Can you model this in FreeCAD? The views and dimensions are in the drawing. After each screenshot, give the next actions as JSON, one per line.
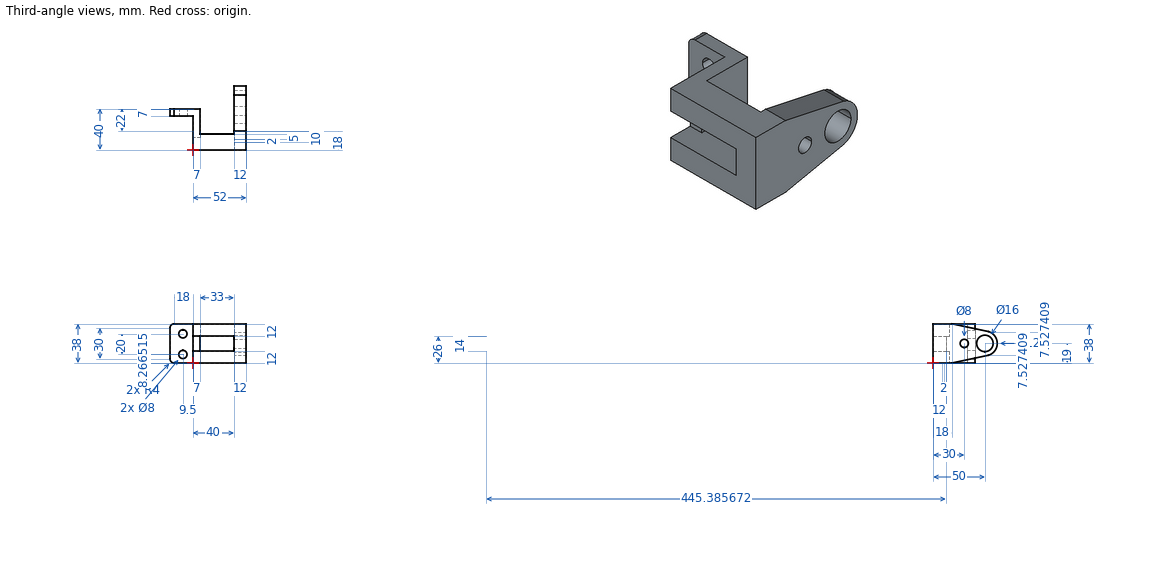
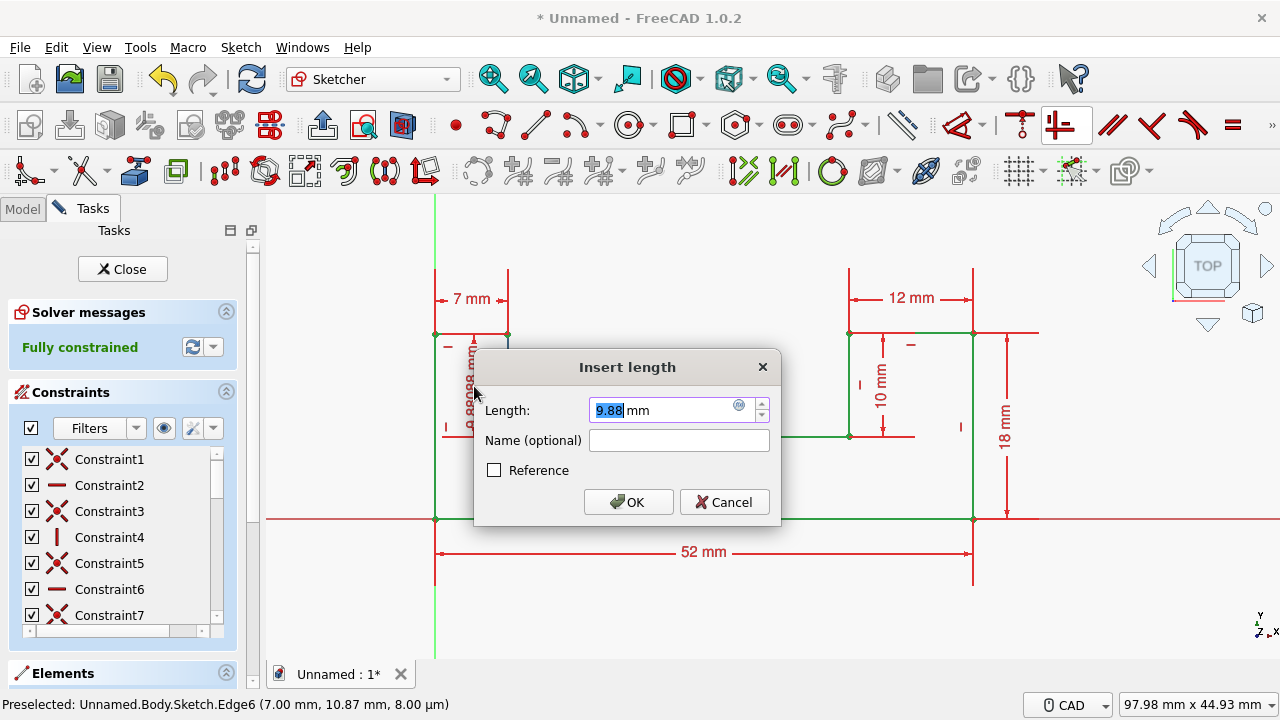
{"action": "type", "text": "10"}
{"action": "key", "text": "Return"}
{"action": "key", "text": "Escape"}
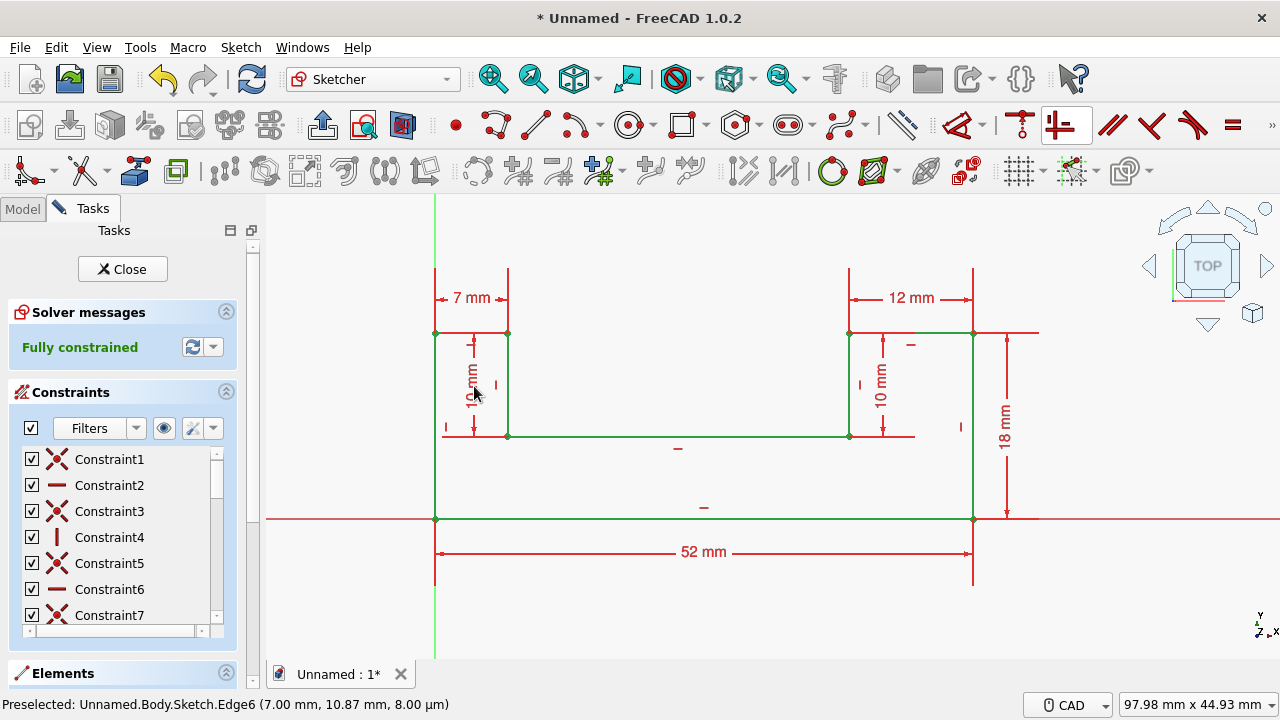
{"action": "left_click", "coordinate": [123, 269]}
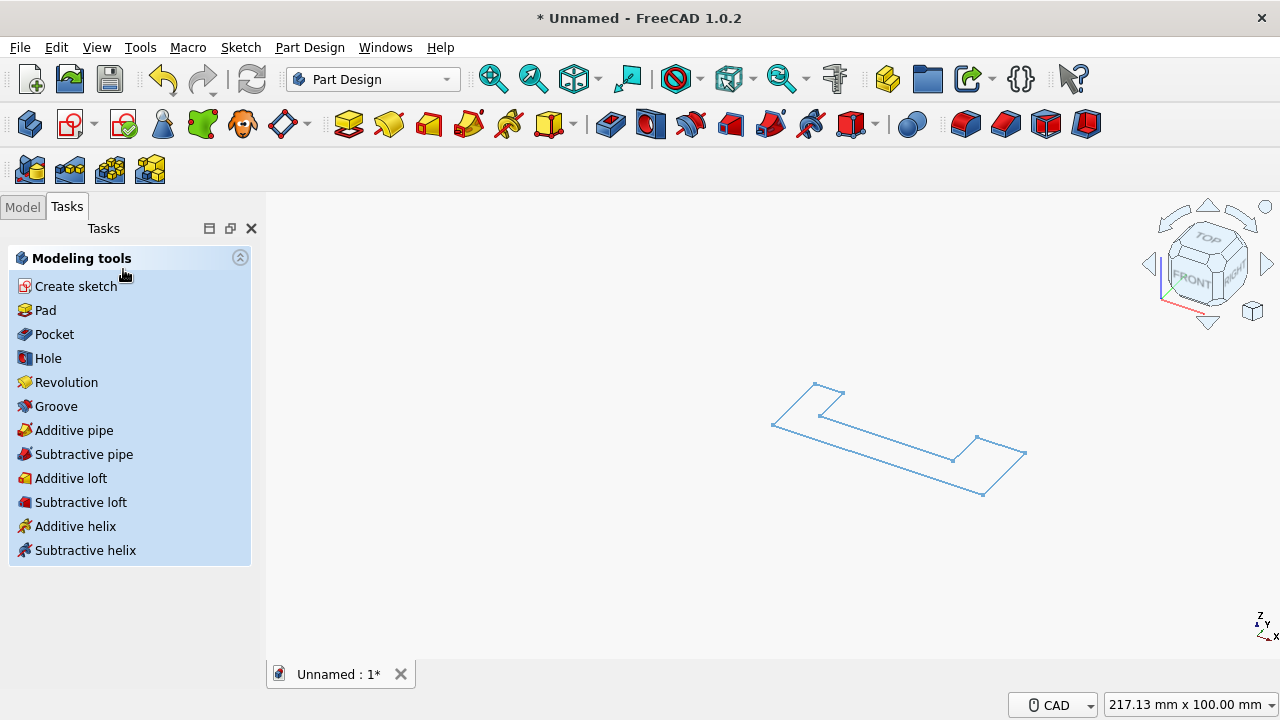
{"action": "left_click", "coordinate": [350, 124]}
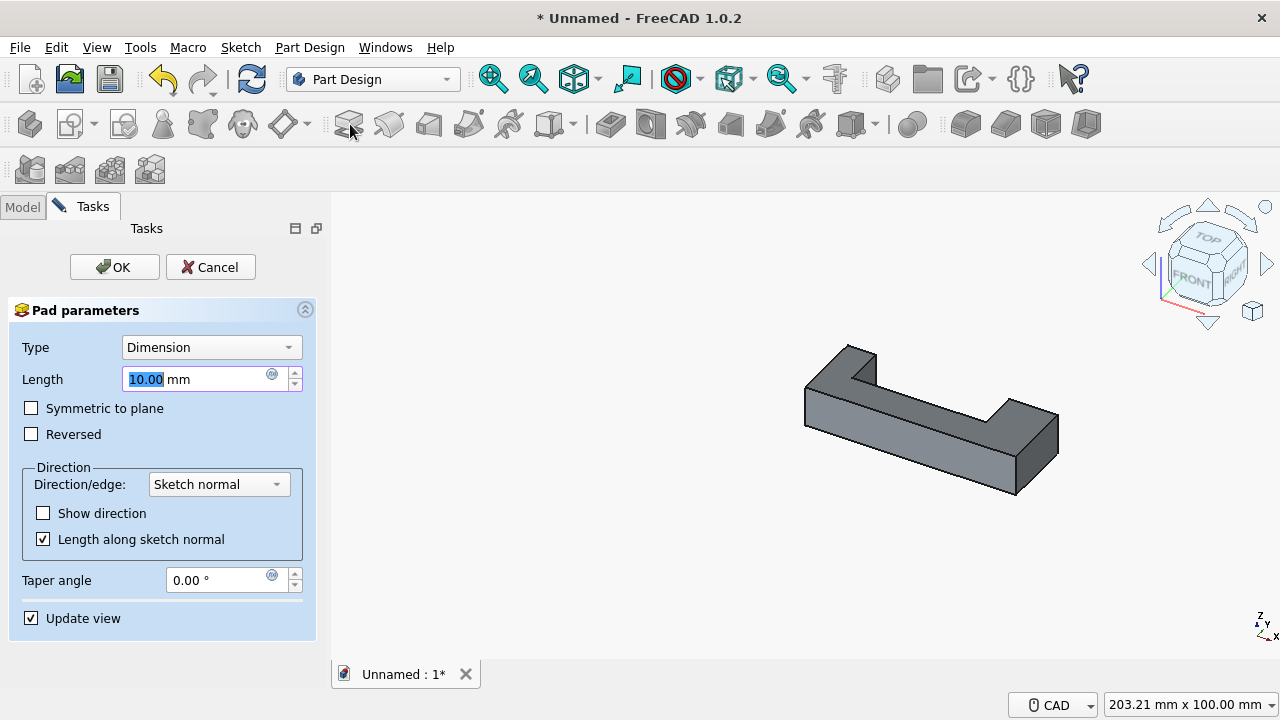
{"action": "type", "text": "38"}
{"action": "key", "text": "Tab"}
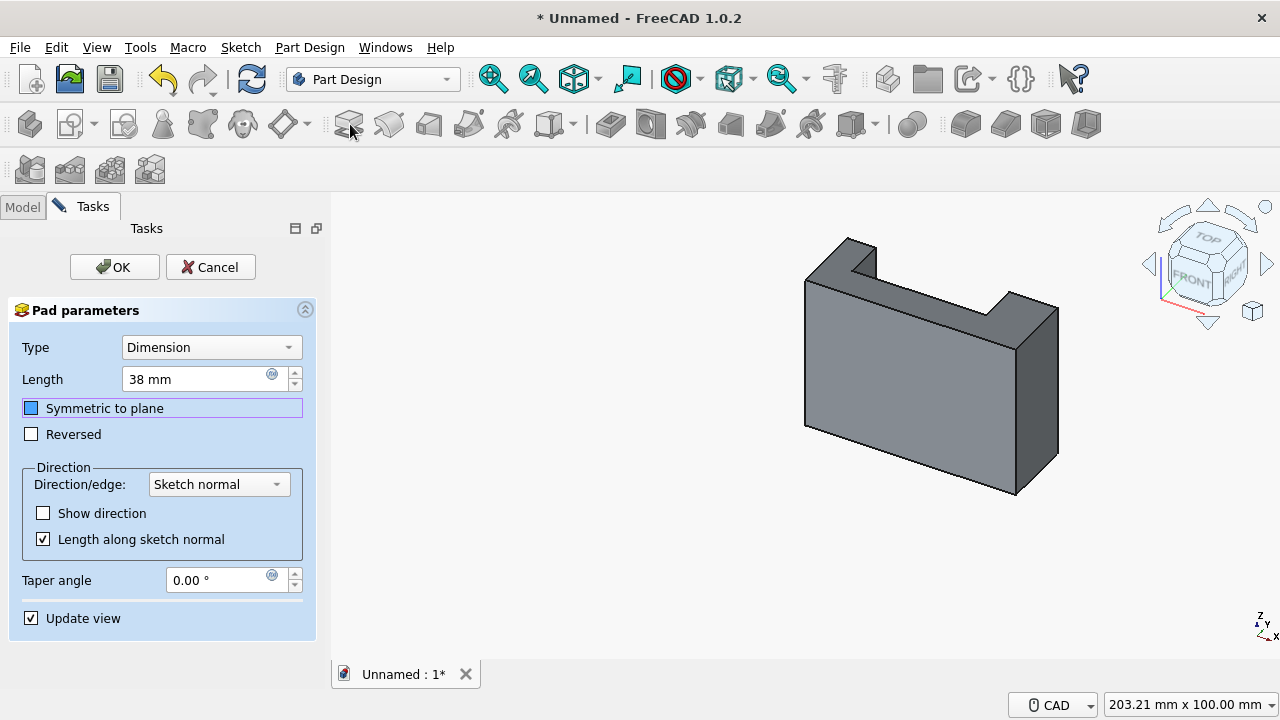
{"action": "left_click", "coordinate": [115, 267]}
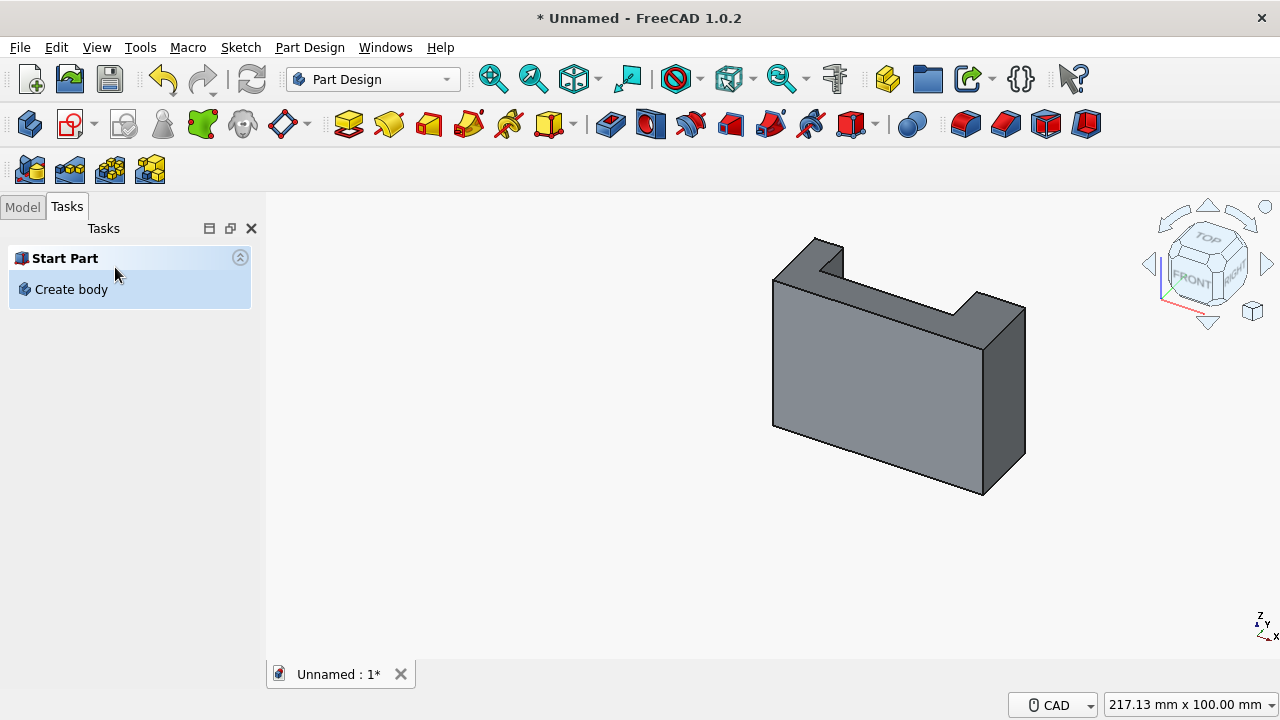
{"action": "left_click", "coordinate": [1004, 380]}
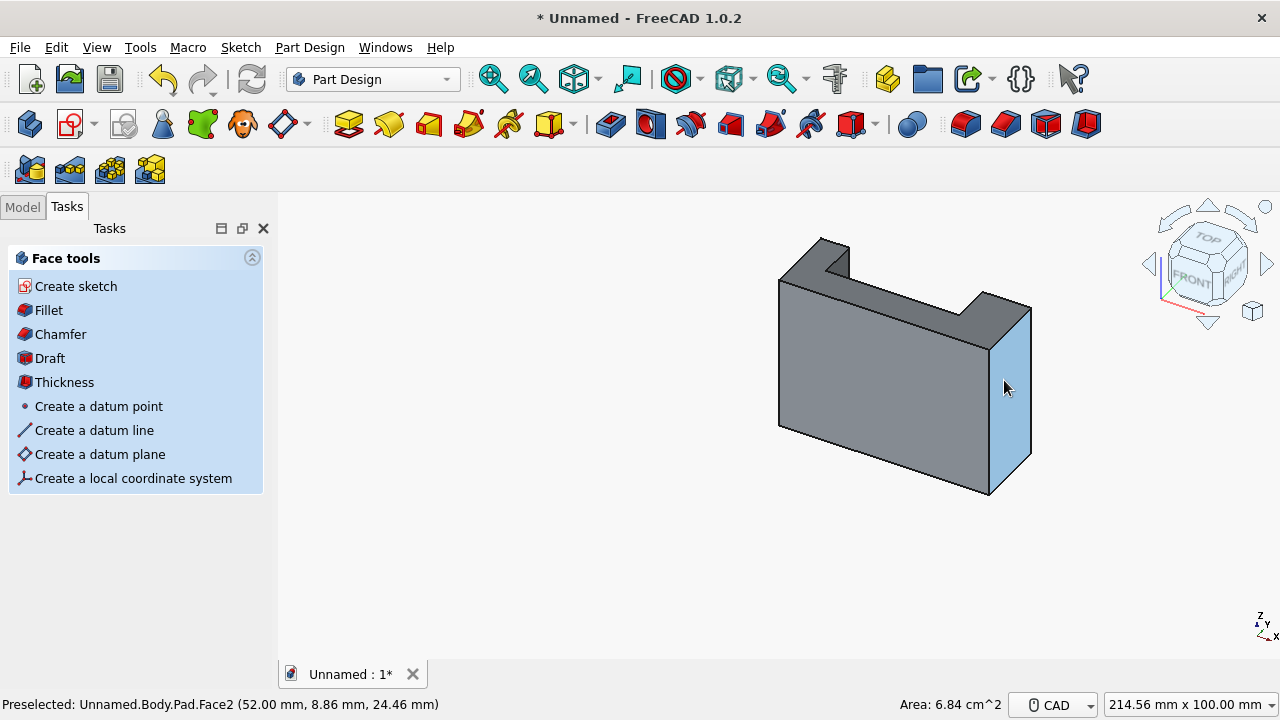
{"action": "left_click", "coordinate": [70, 124]}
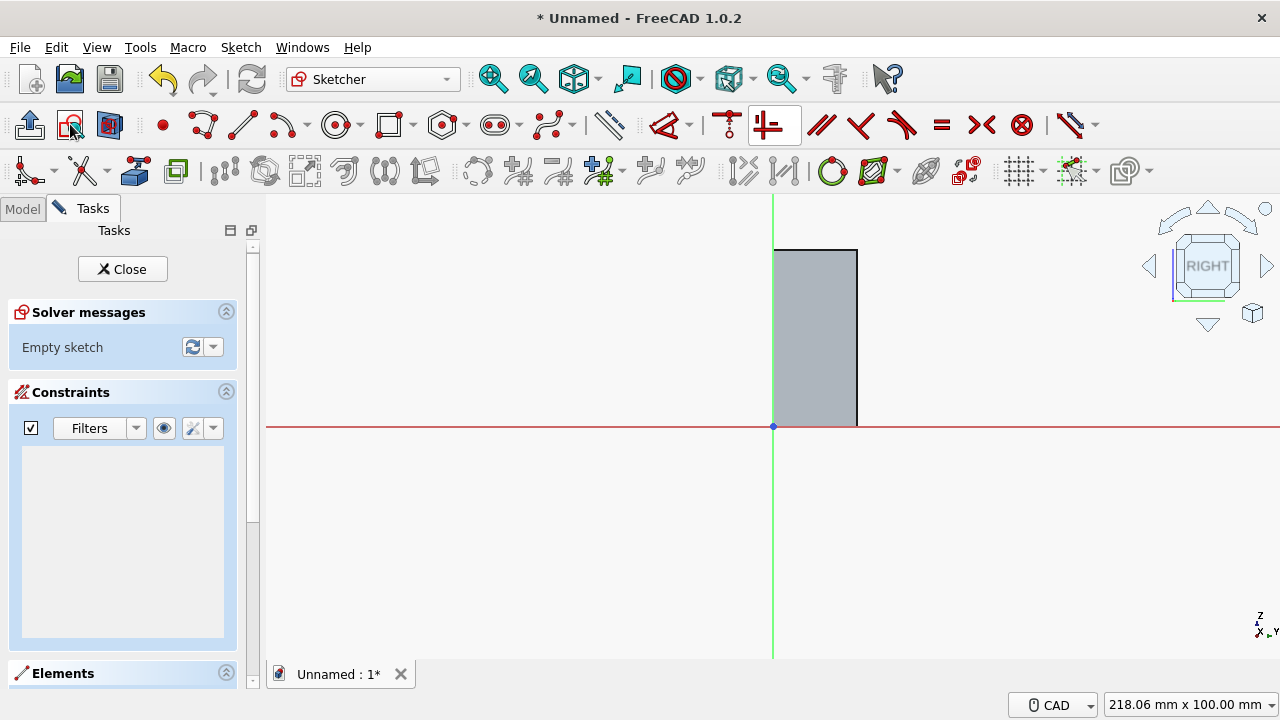
{"action": "scroll", "coordinate": [1115, 222], "scroll_direction": "up", "scroll_amount": 2}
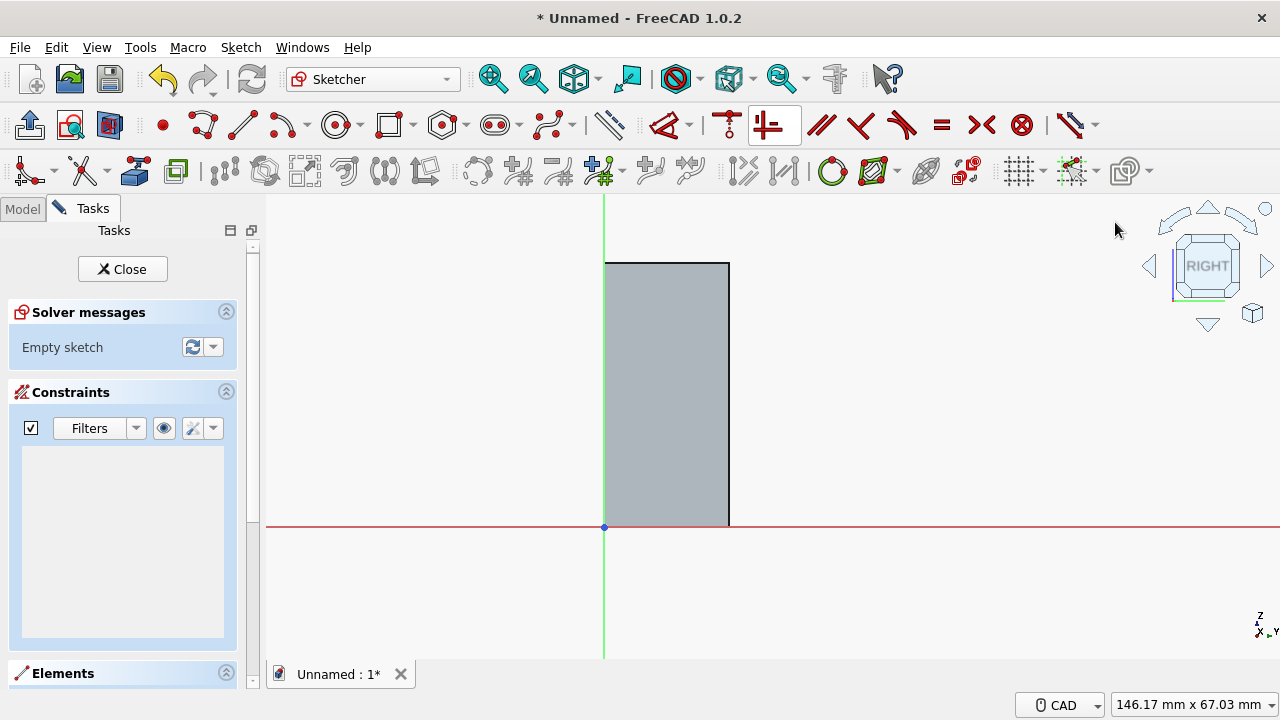
{"action": "left_click", "coordinate": [204, 126]}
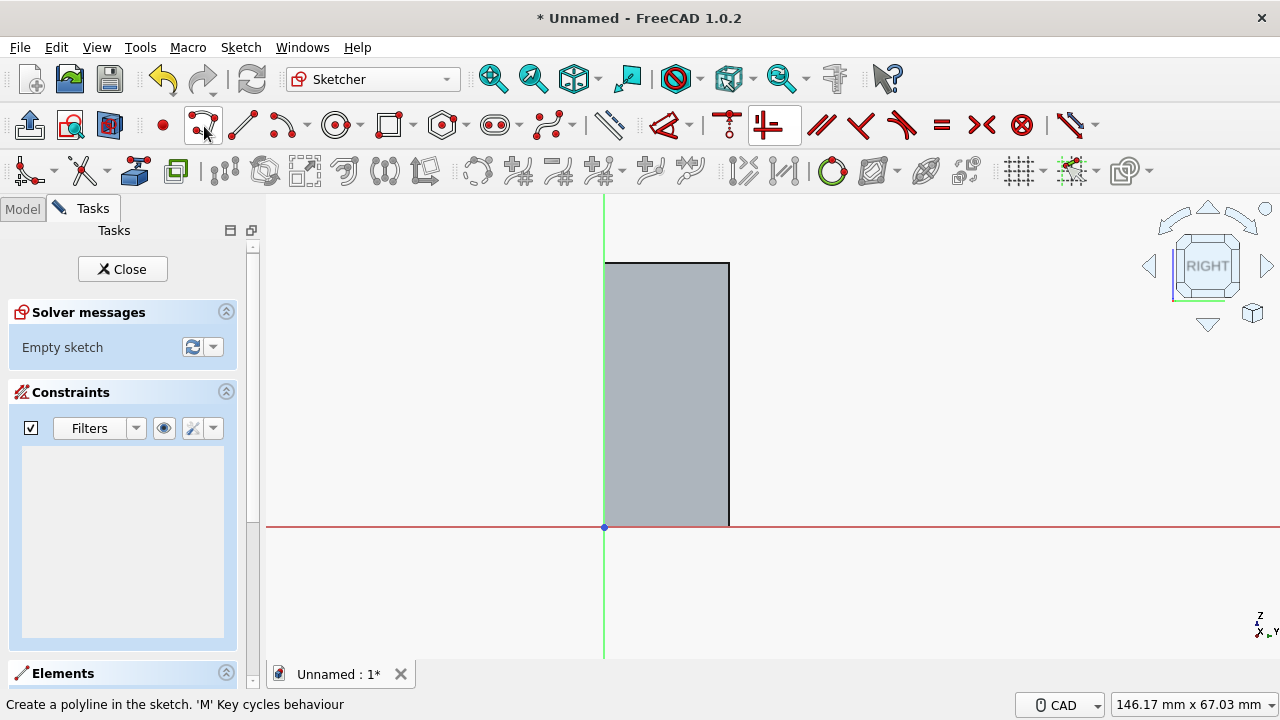
{"action": "left_click", "coordinate": [976, 316]}
{"action": "left_click", "coordinate": [729, 263]}
{"action": "left_click", "coordinate": [729, 527]}
{"action": "left_click", "coordinate": [976, 475]}
{"action": "right_click", "coordinate": [976, 475]}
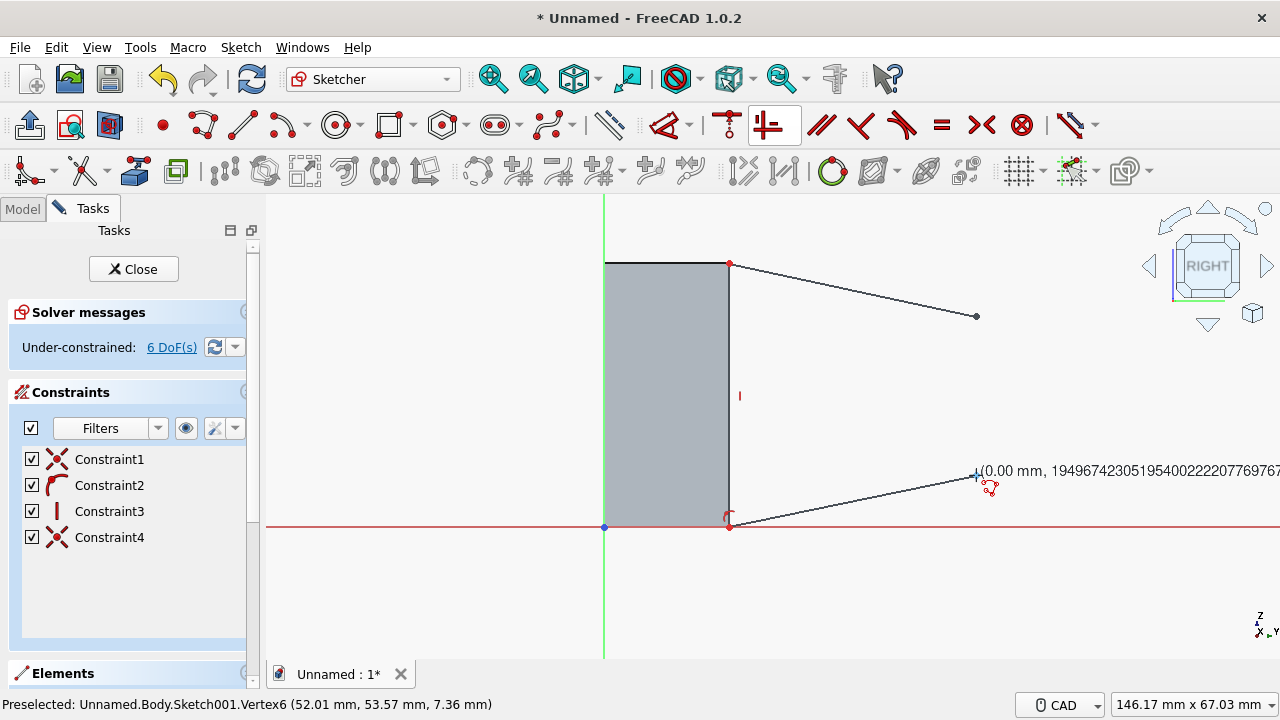
{"action": "left_click", "coordinate": [310, 126]}